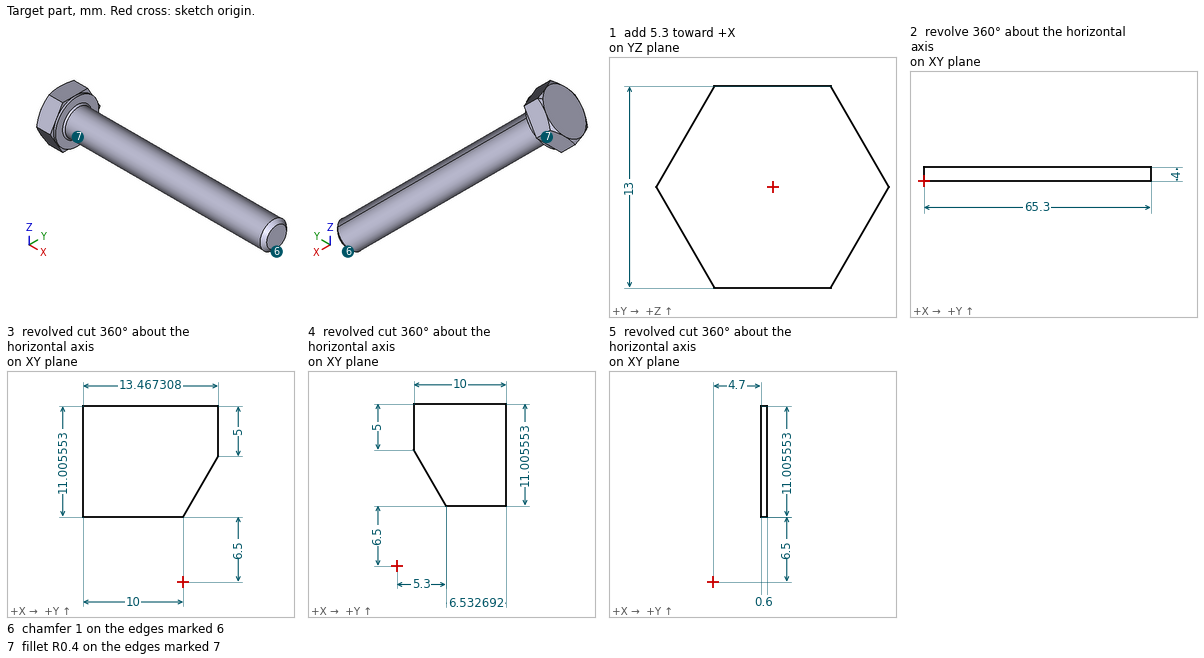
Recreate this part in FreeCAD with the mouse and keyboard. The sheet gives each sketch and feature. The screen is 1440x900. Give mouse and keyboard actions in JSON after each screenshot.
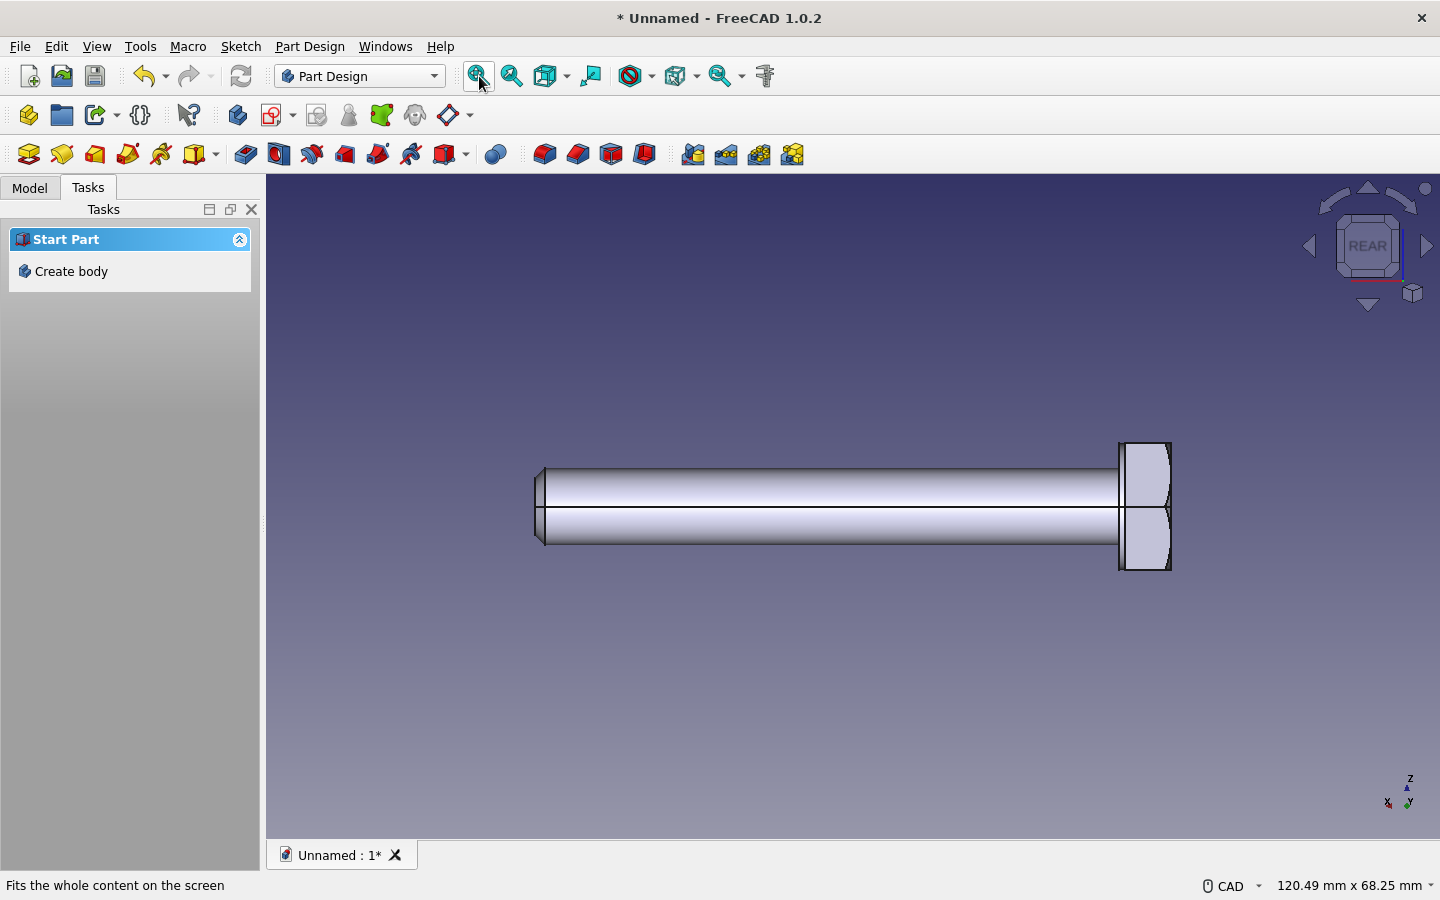
{"action": "key", "text": "6"}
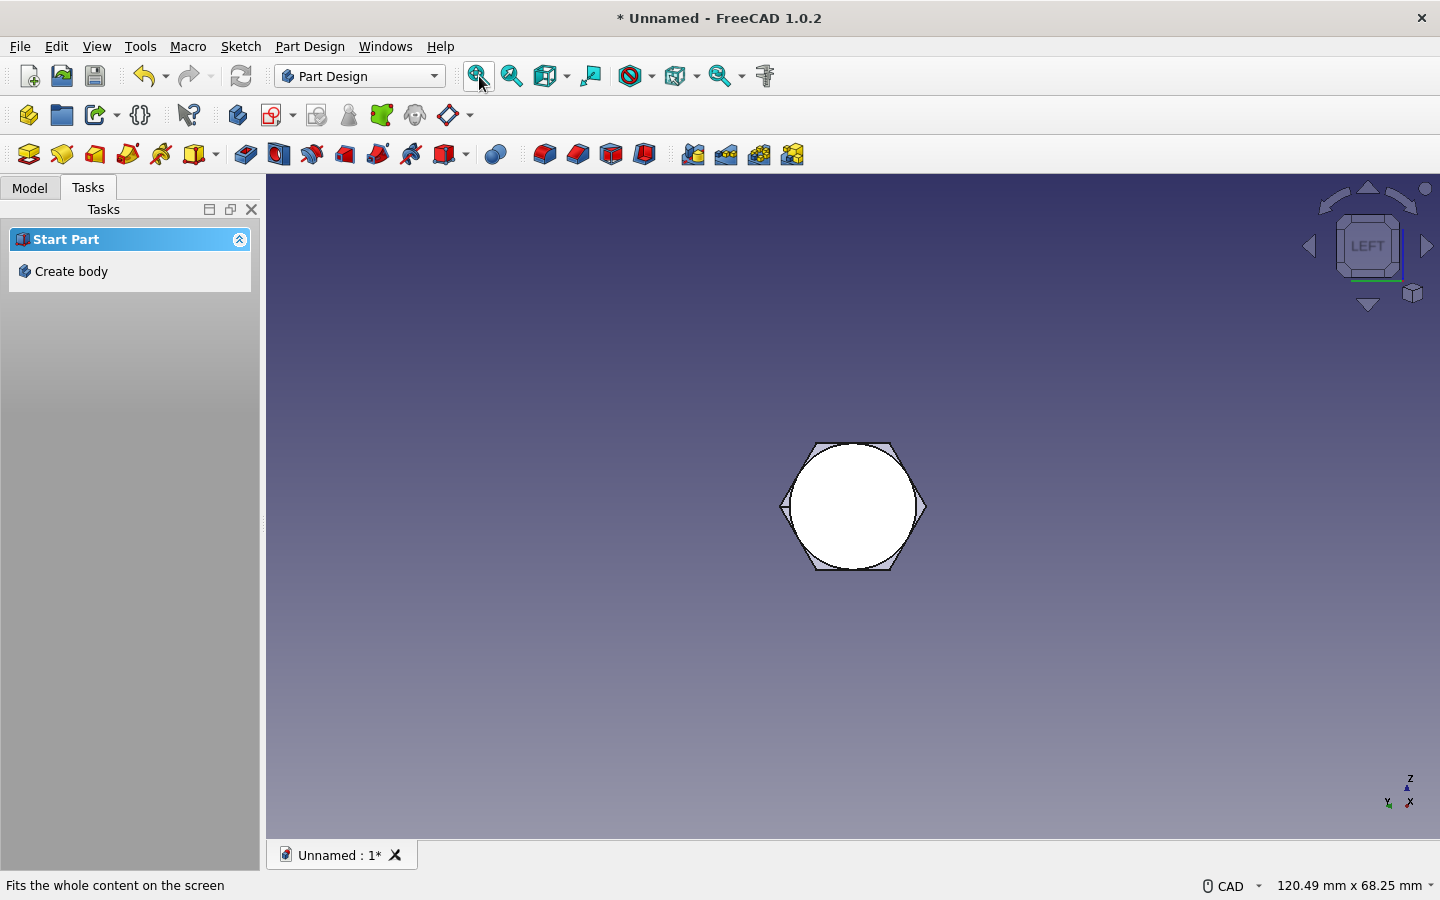
{"action": "left_click", "coordinate": [479, 76]}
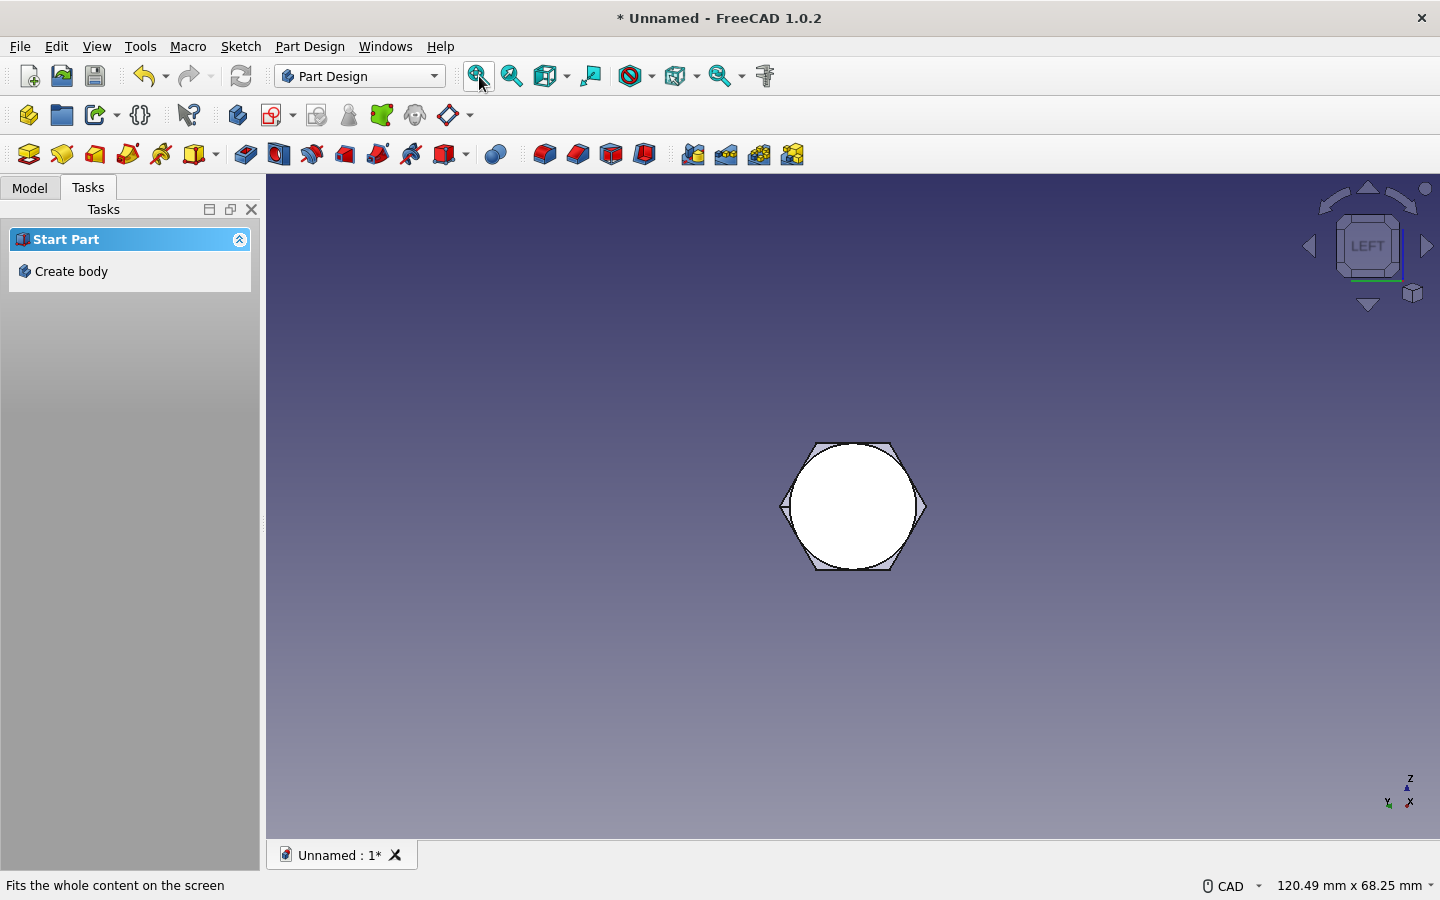
{"action": "key", "text": "v 3"}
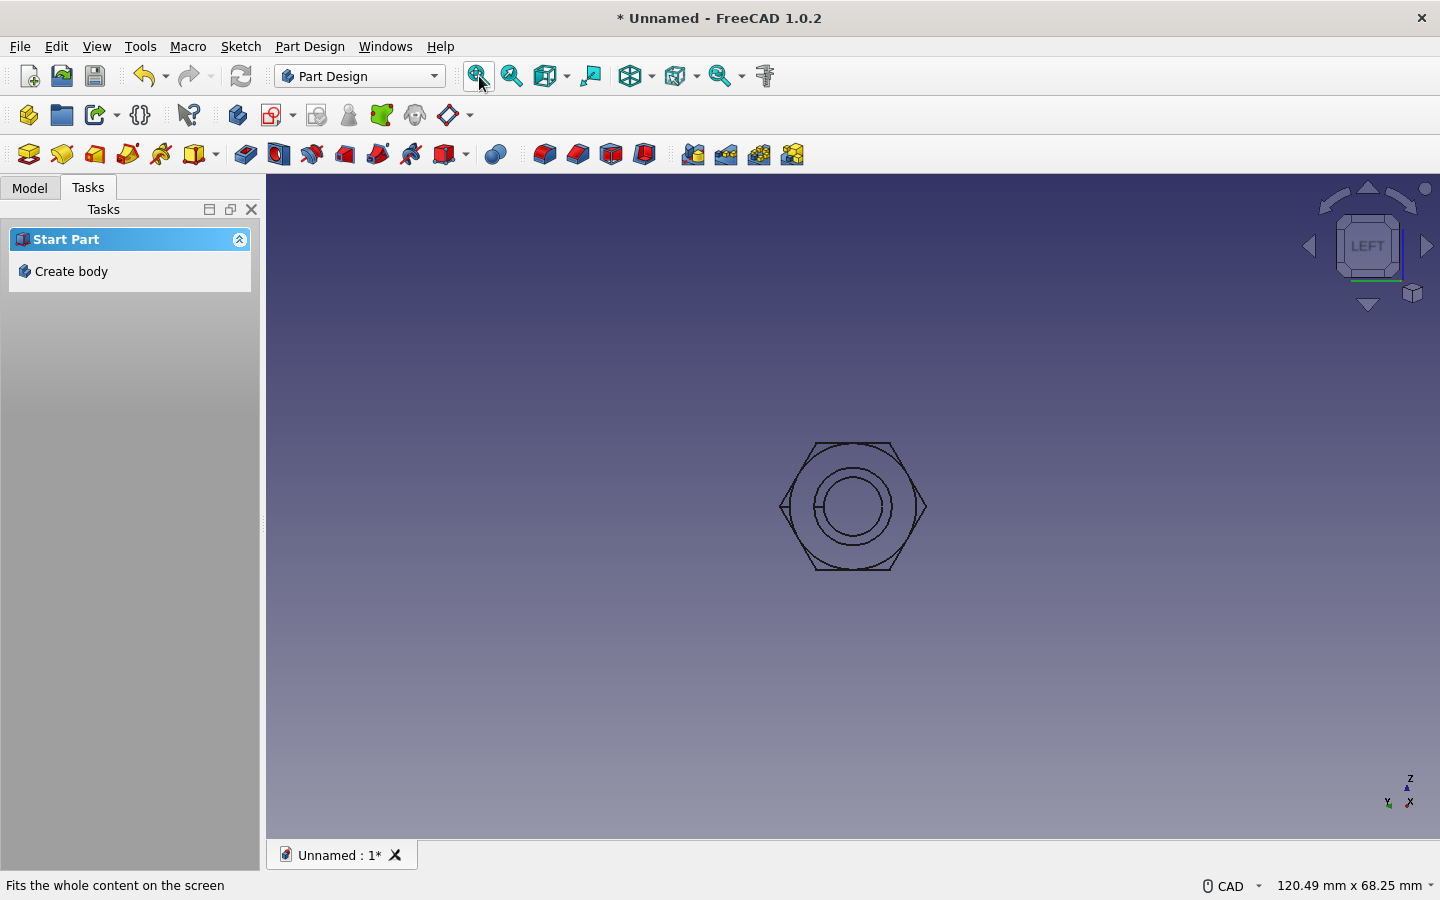
{"action": "key", "text": "0"}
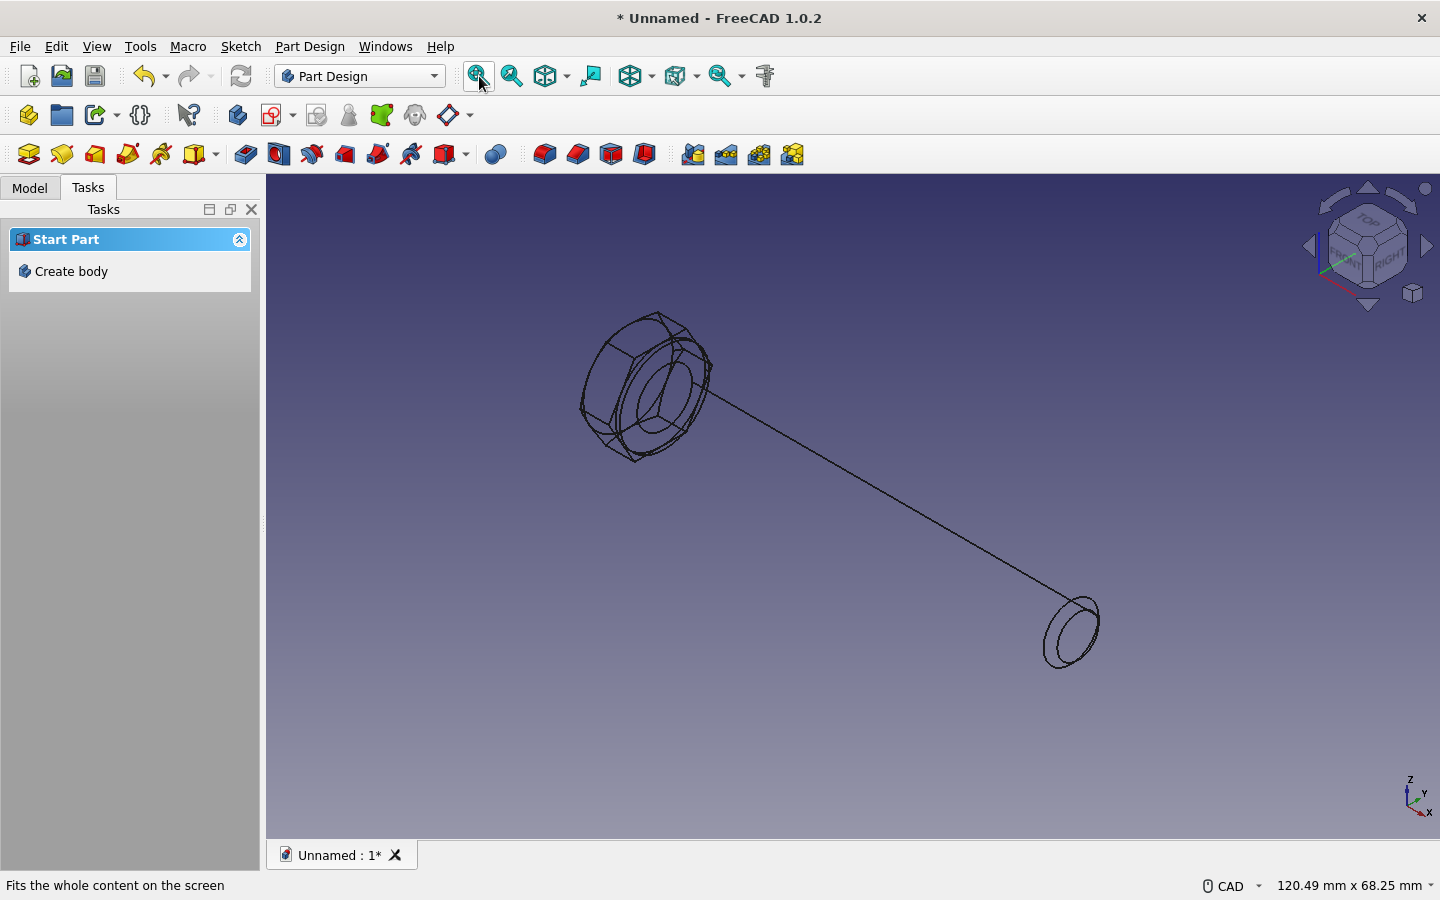
{"action": "left_click", "coordinate": [637, 413]}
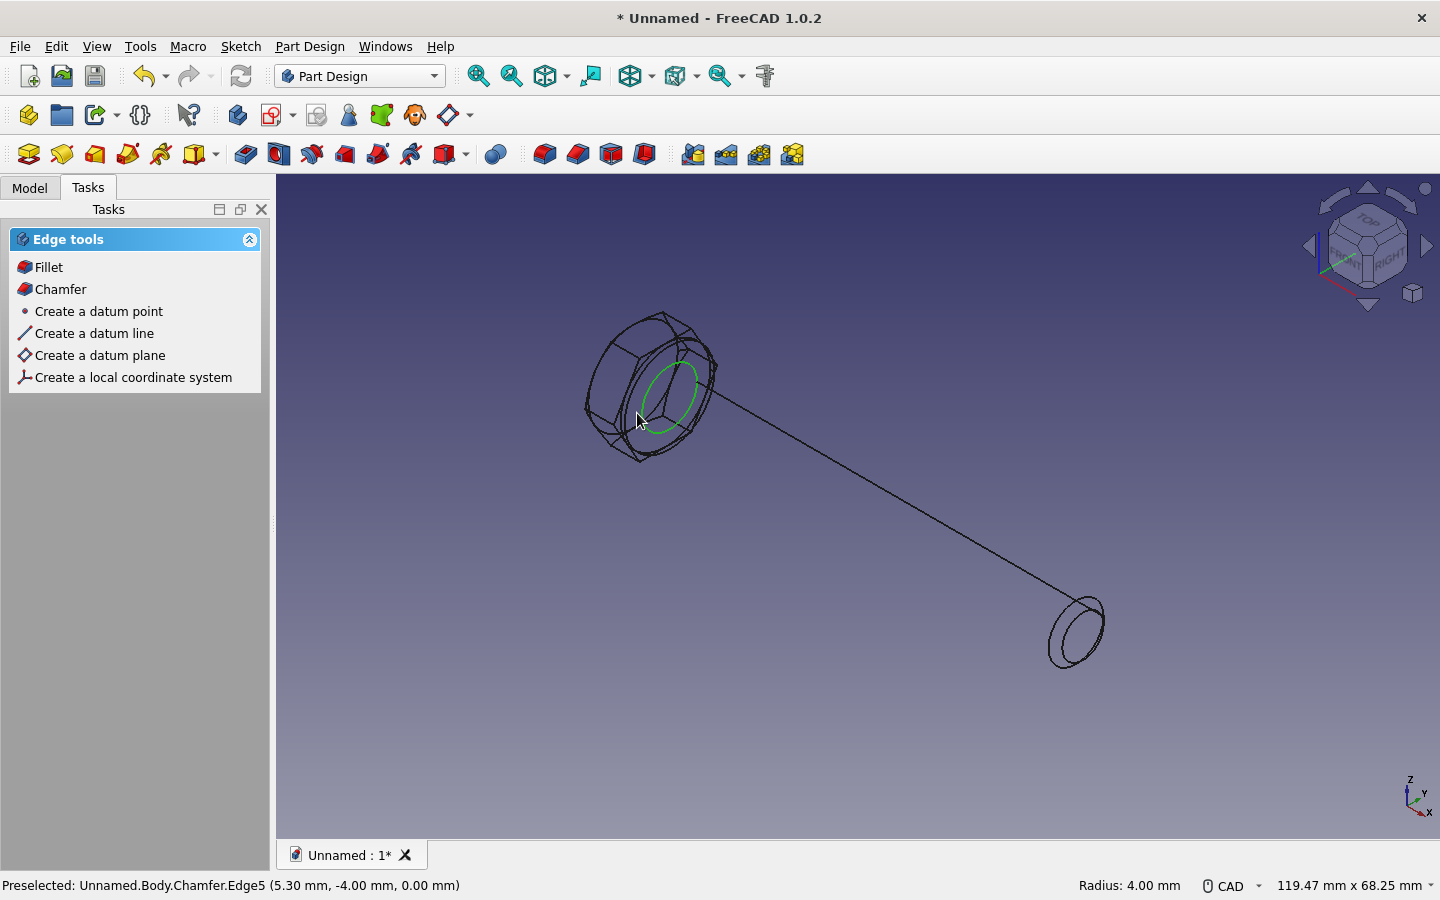
{"action": "key", "text": "v 1"}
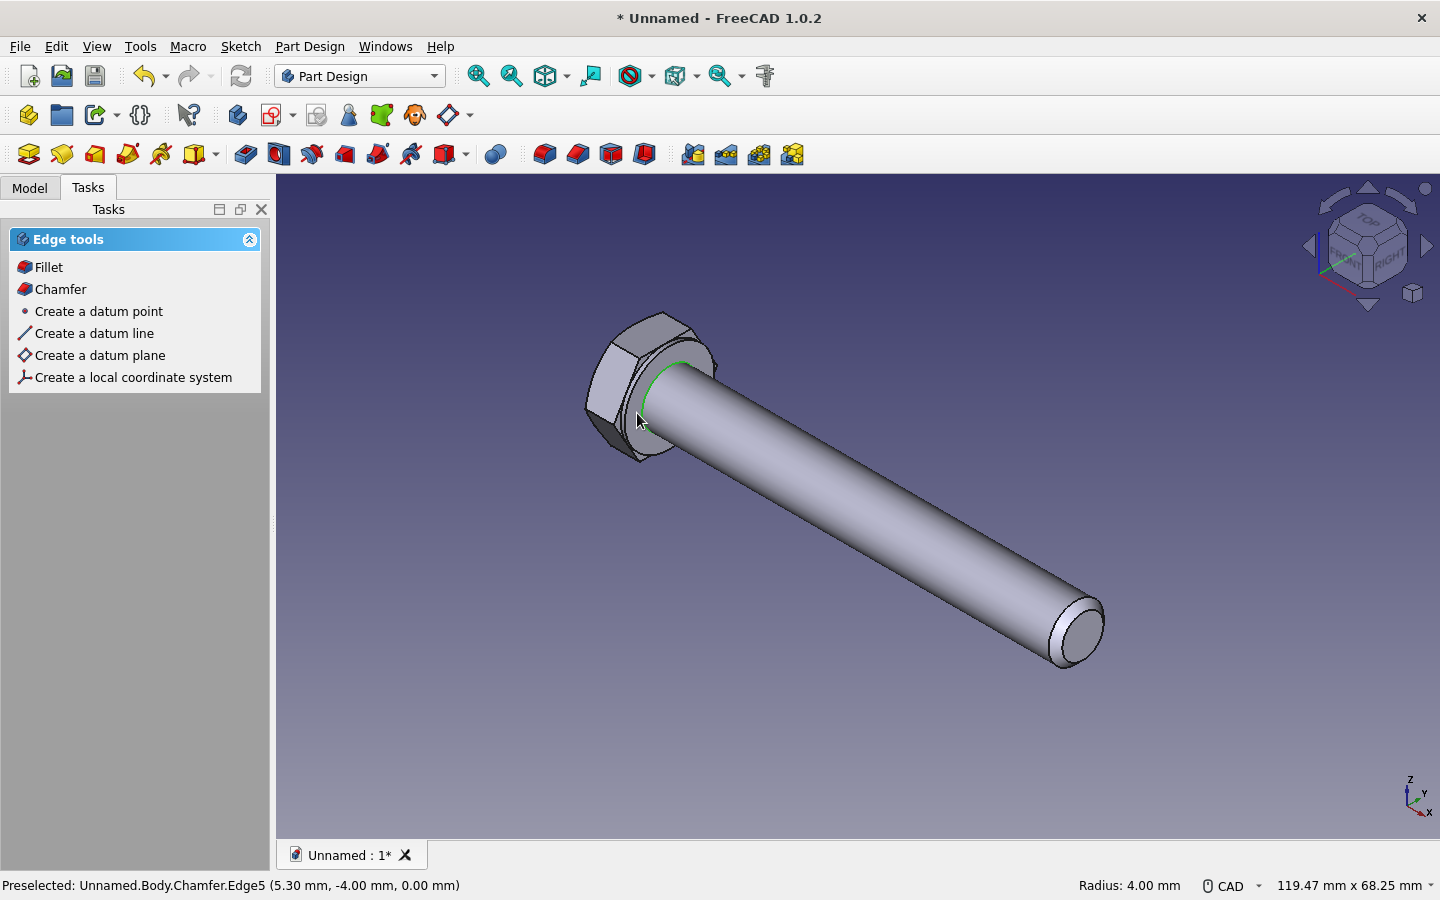
{"action": "left_click", "coordinate": [545, 154]}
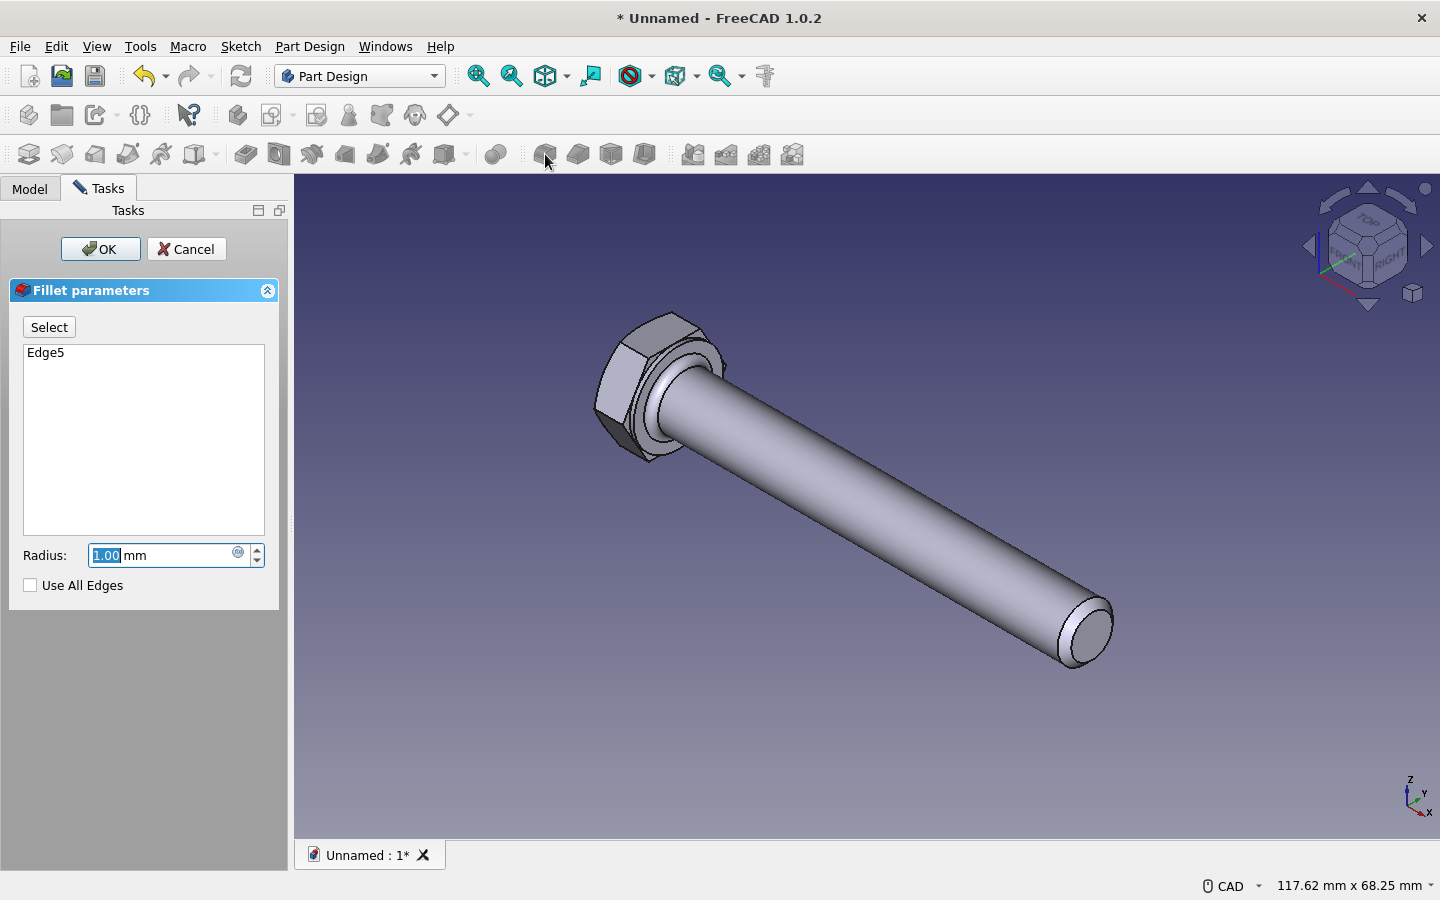
{"action": "type", "text": "0.4"}
{"action": "key", "text": "Tab"}